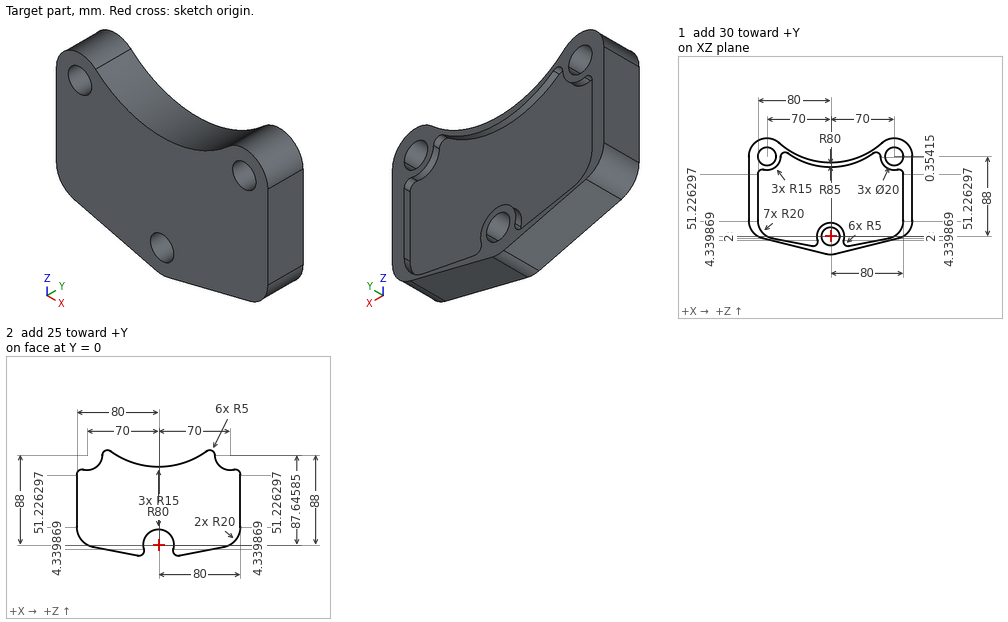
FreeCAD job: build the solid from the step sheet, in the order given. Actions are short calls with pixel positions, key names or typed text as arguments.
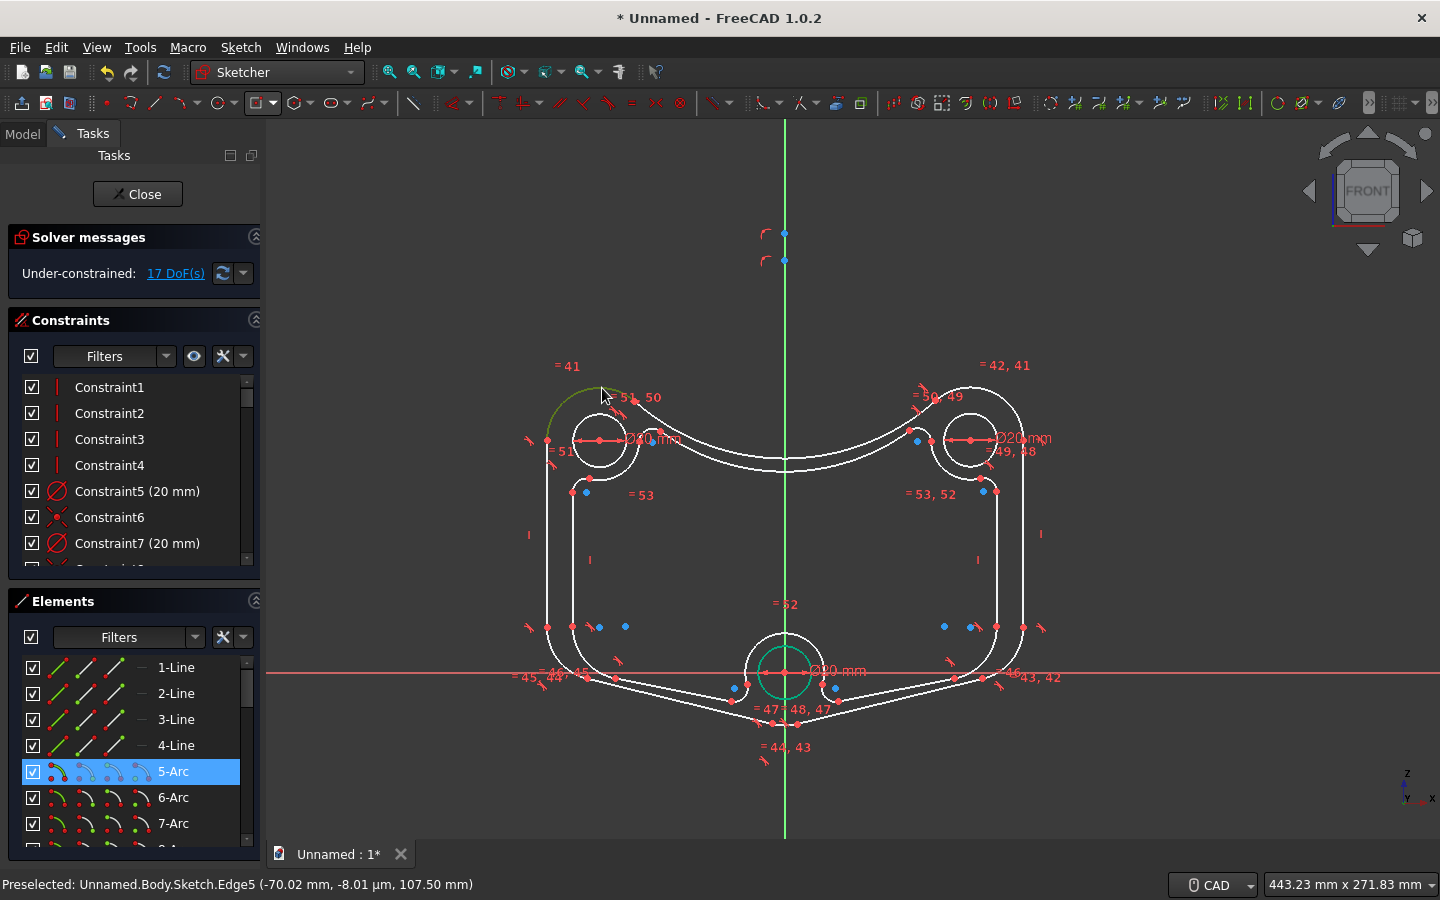
key(k)
key(r)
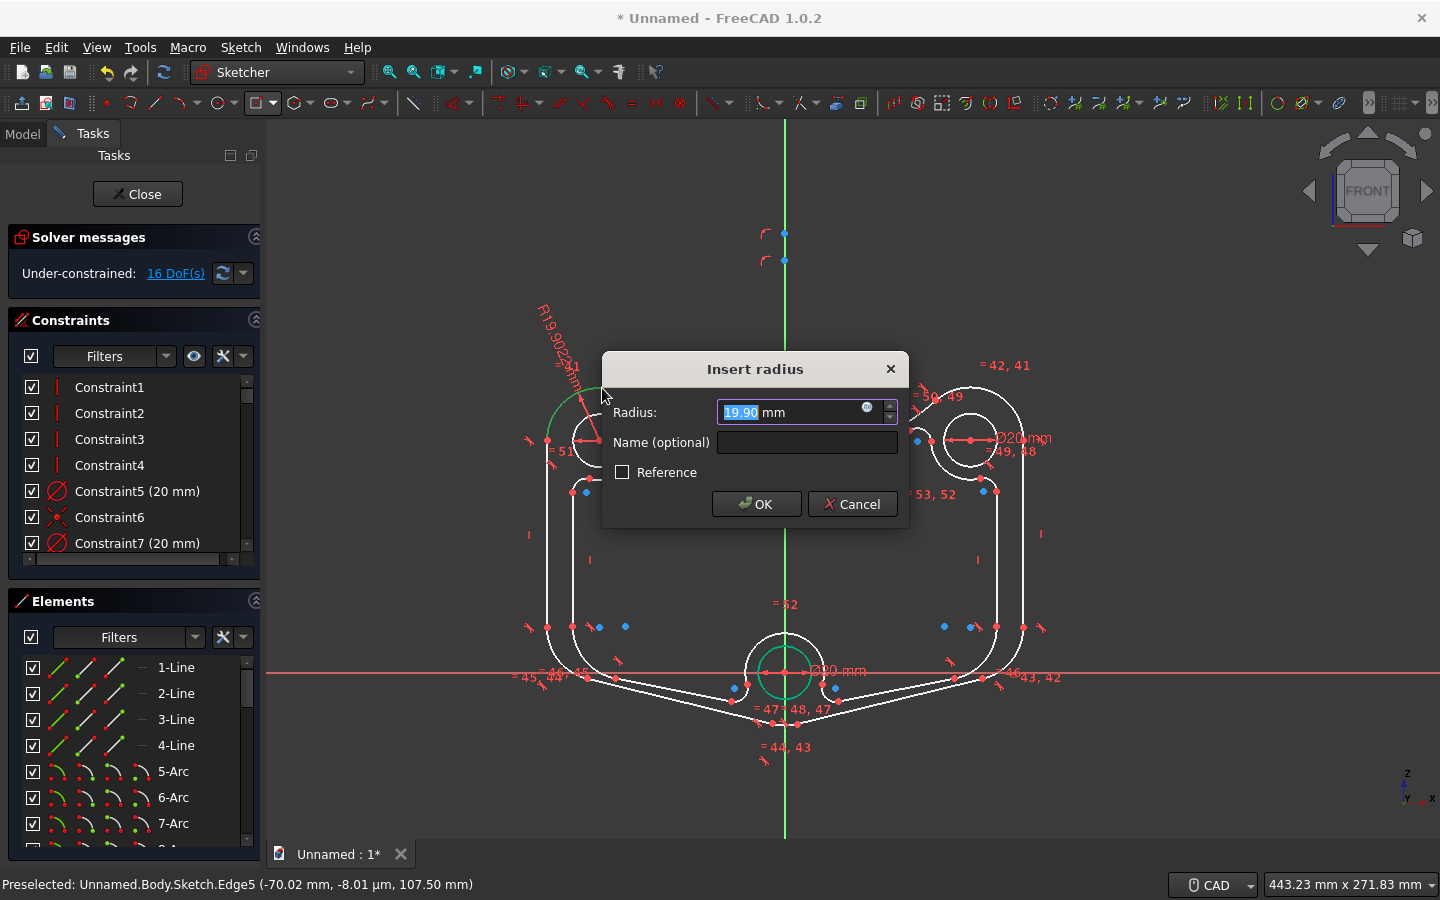
text(20)
key(Return)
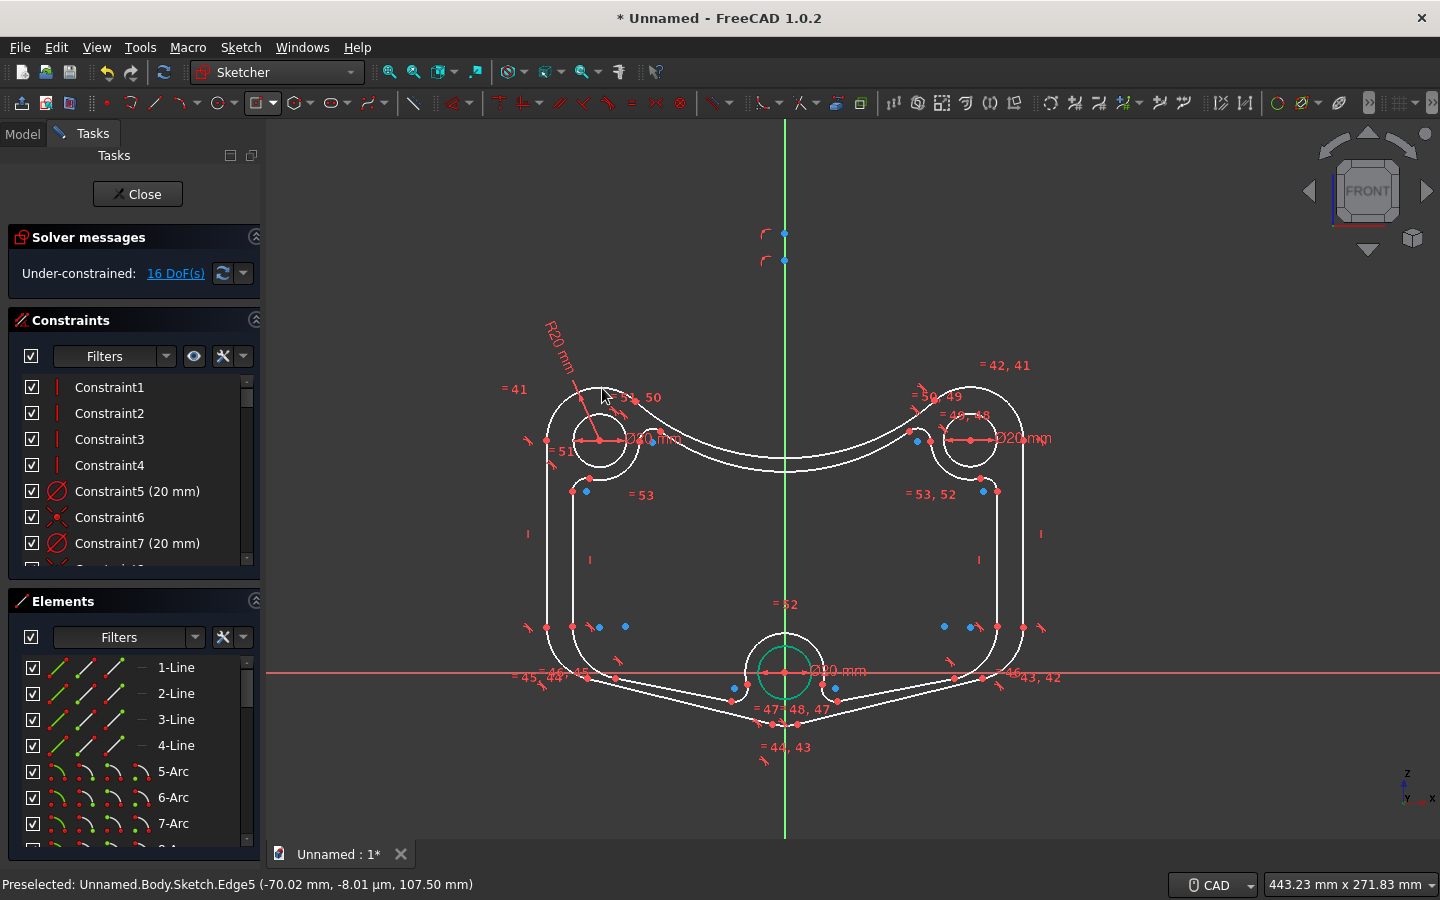
click(720, 449)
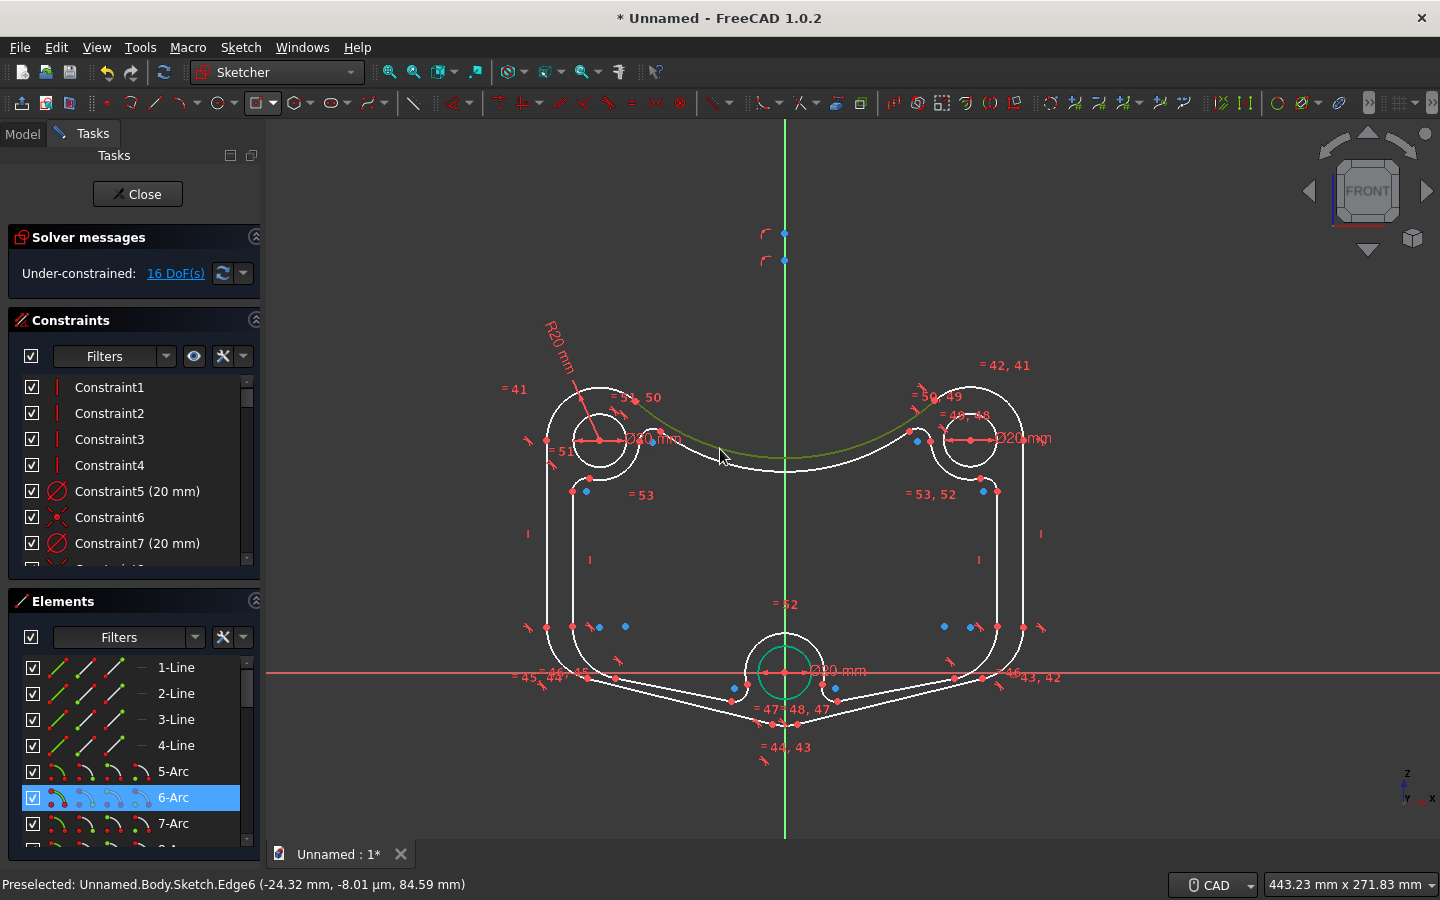
click(472, 104)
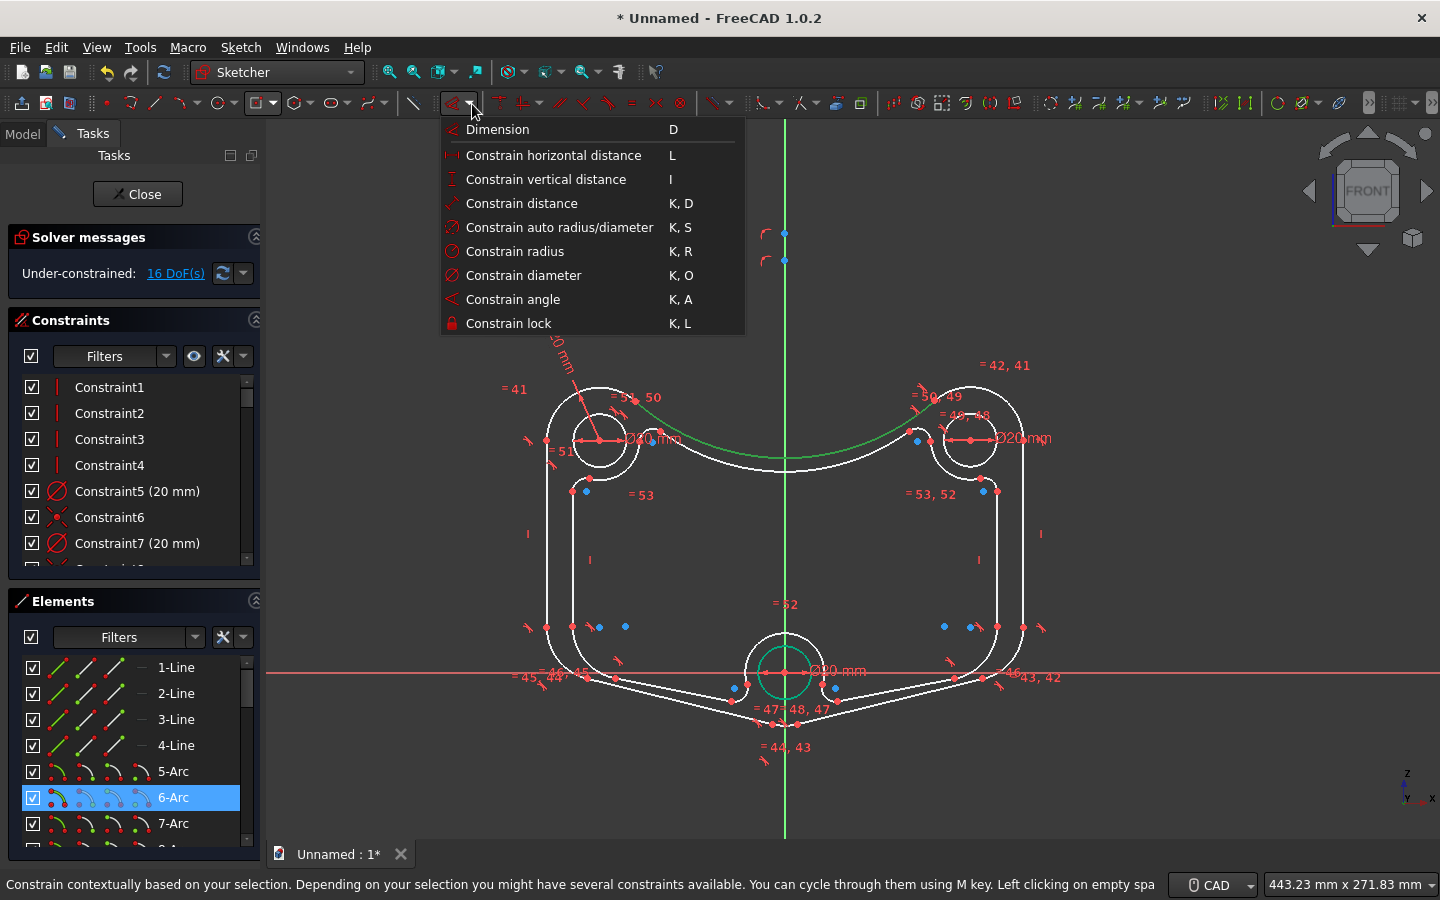
click(593, 251)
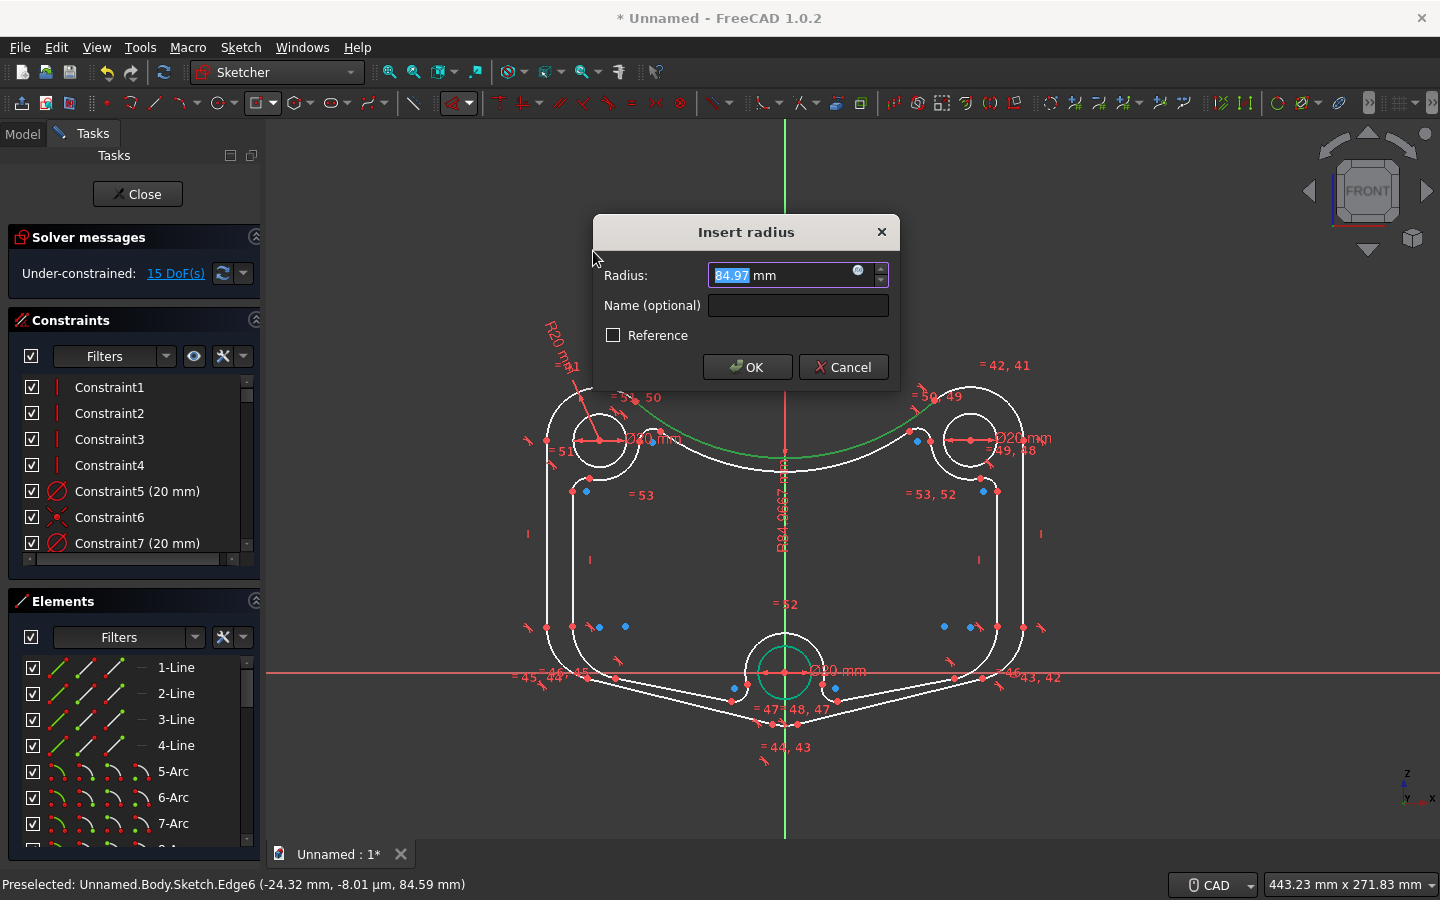
text(85)
key(Return)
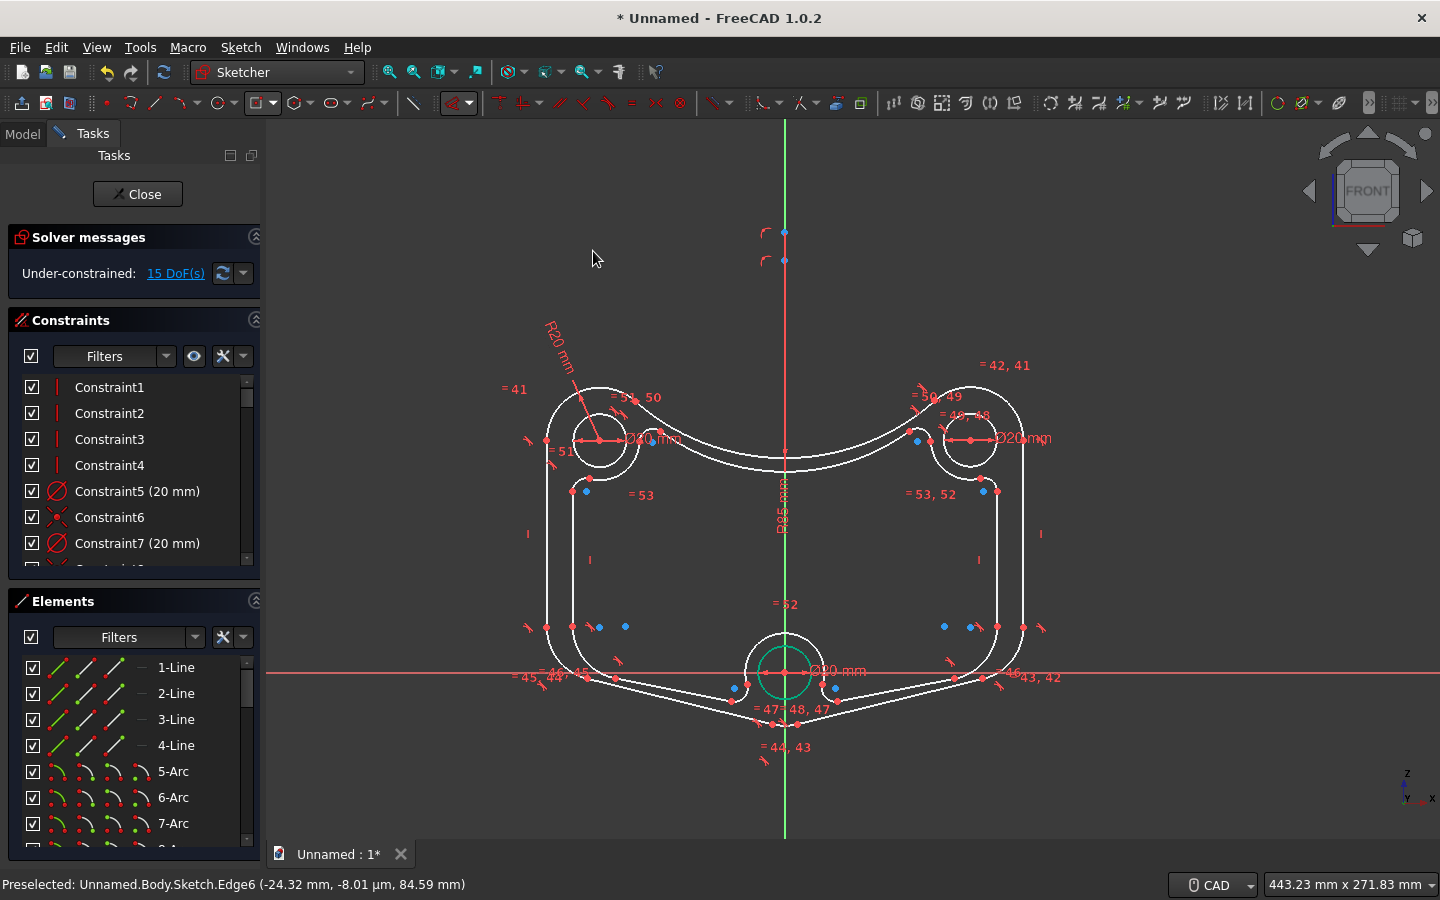
scroll(744, 697, up, 6)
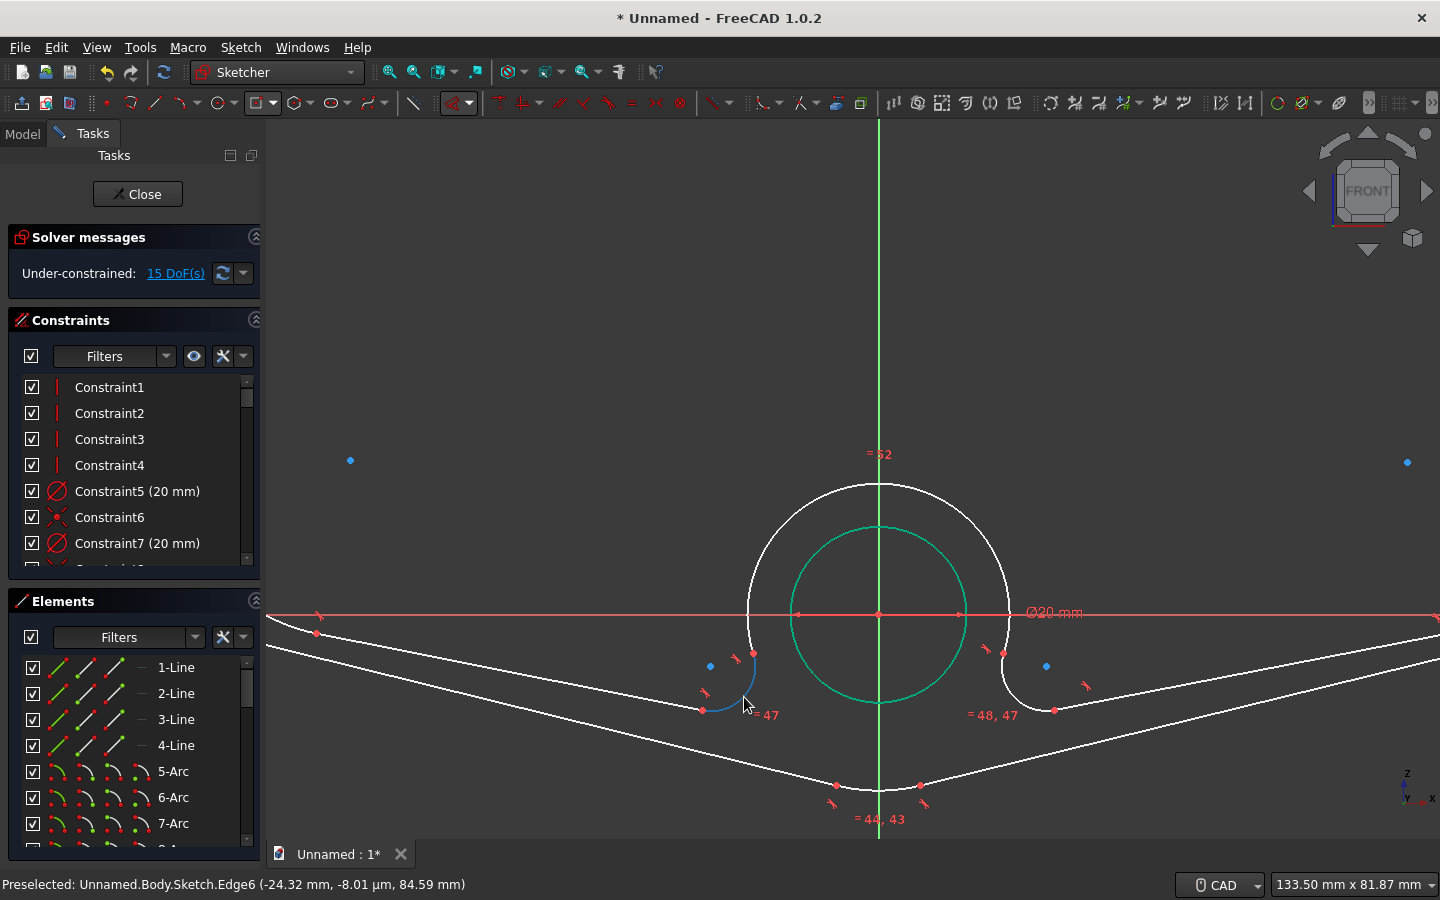
click(744, 696)